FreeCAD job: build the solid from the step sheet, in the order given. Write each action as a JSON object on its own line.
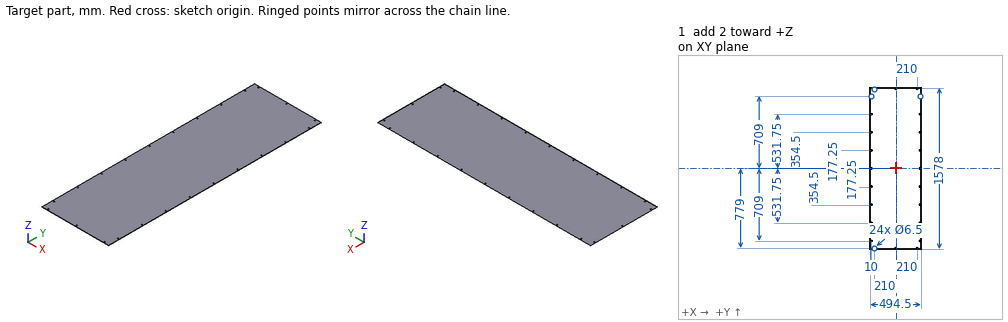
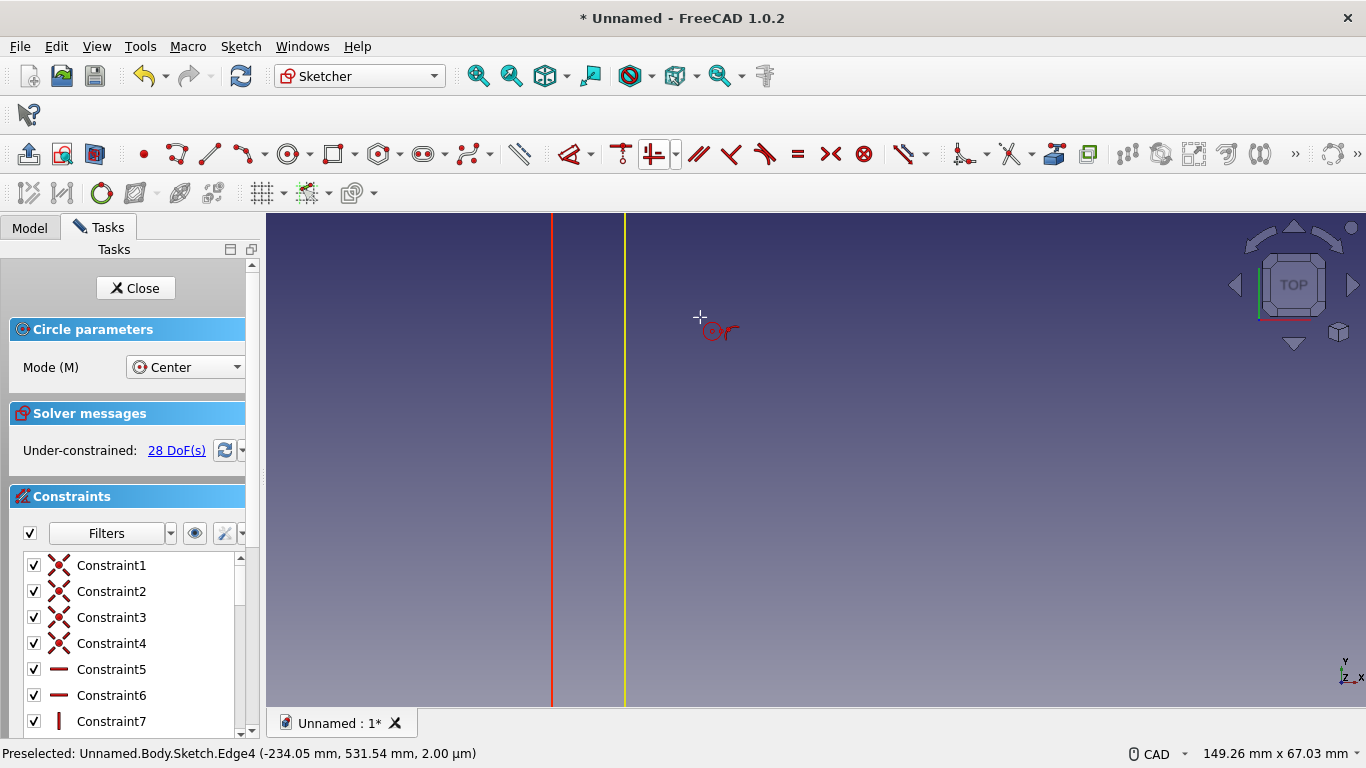
{"action": "scroll", "coordinate": [700, 317], "scroll_direction": "down", "scroll_amount": 18}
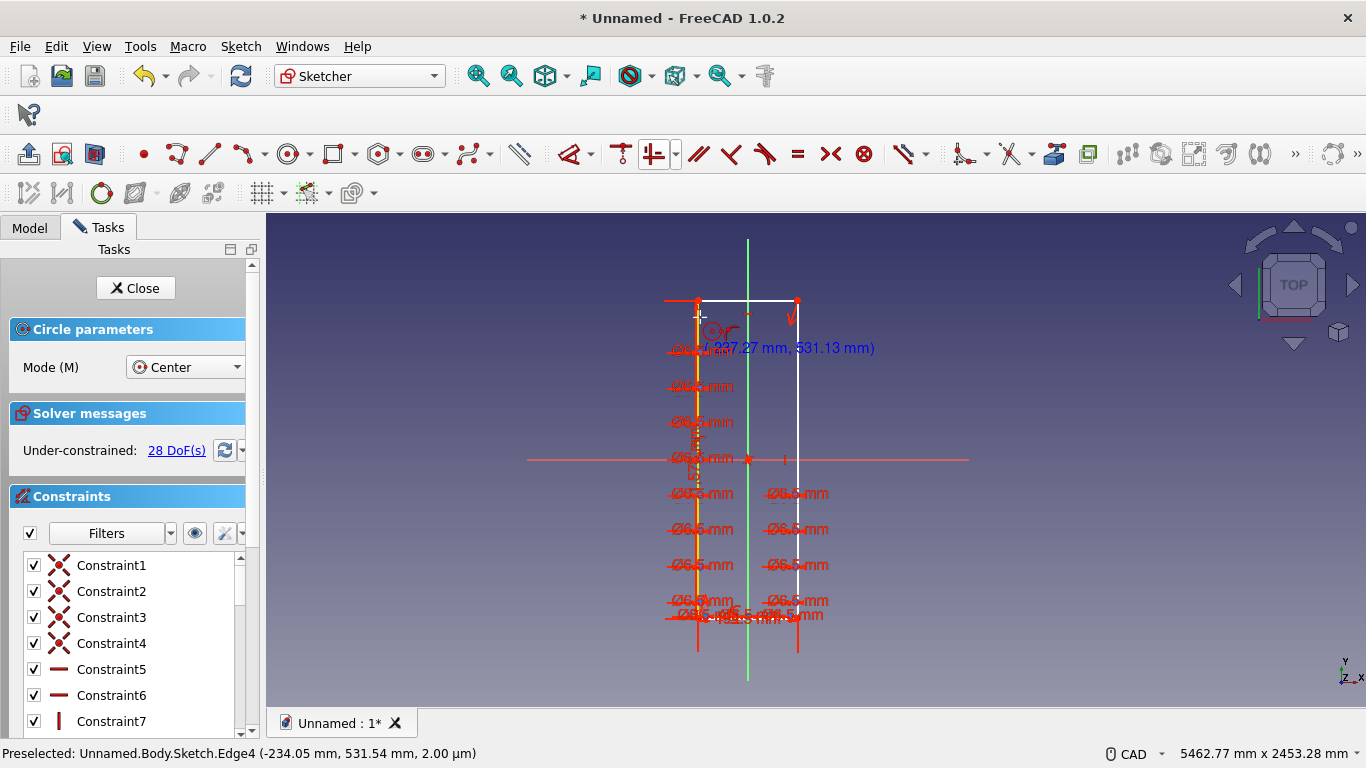
{"action": "scroll", "coordinate": [700, 317], "scroll_direction": "up", "scroll_amount": 11}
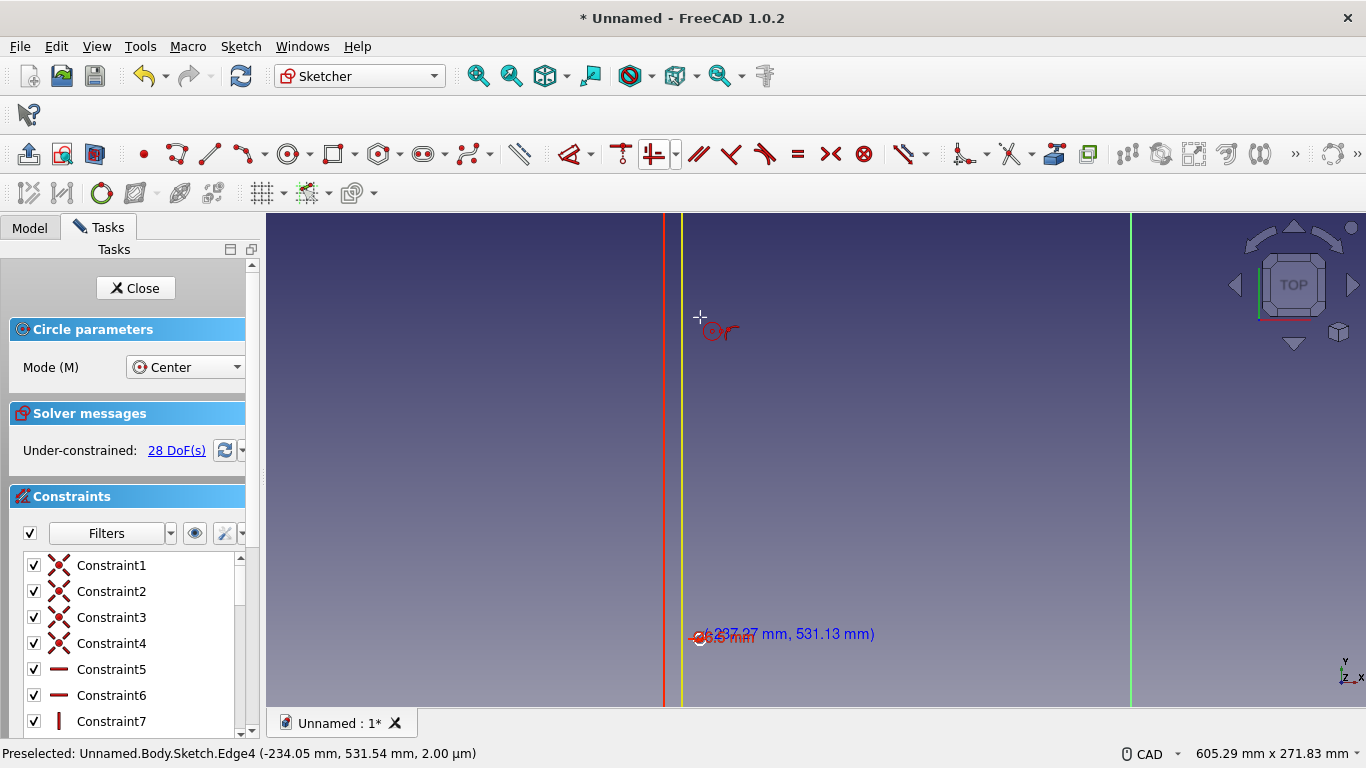
{"action": "left_click", "coordinate": [700, 316]}
{"action": "mouse_move", "coordinate": [704, 312]}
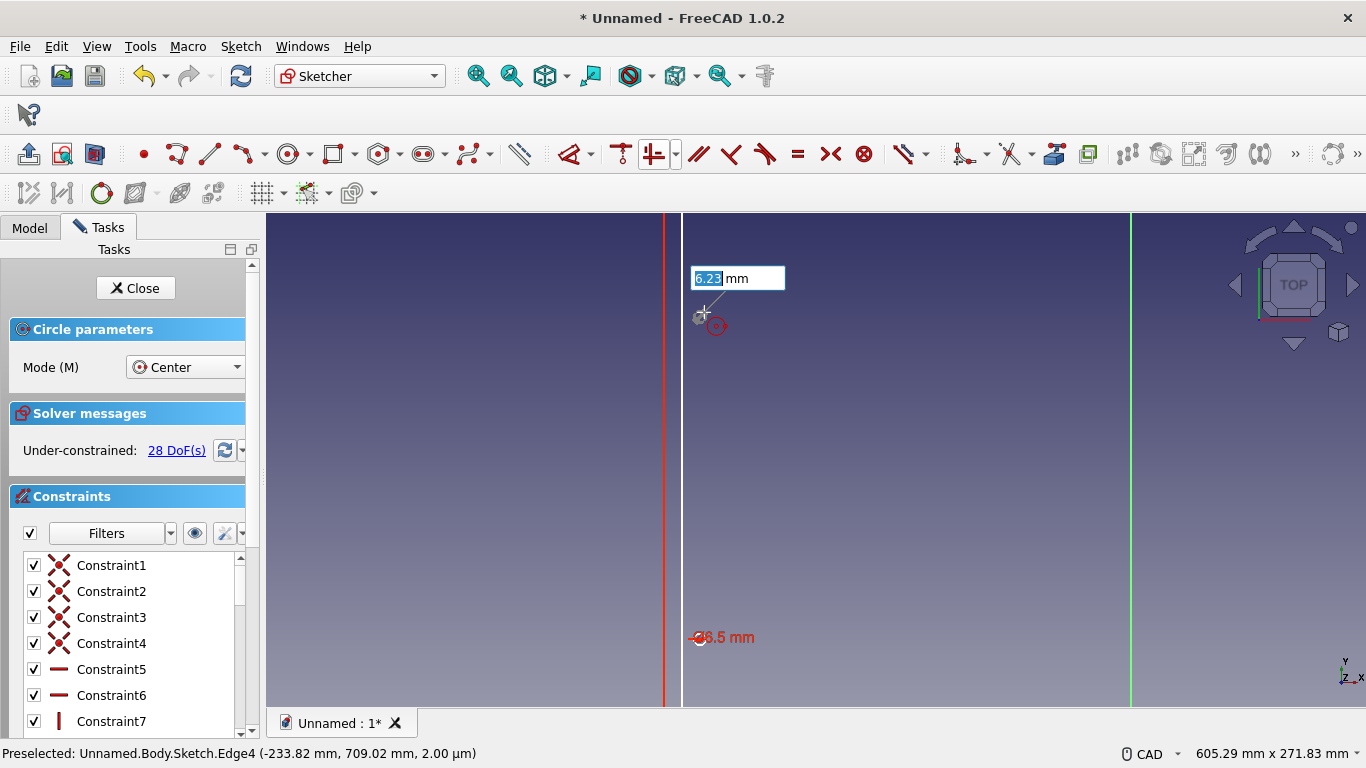
{"action": "type", "text": "6.5"}
{"action": "key", "text": "Return"}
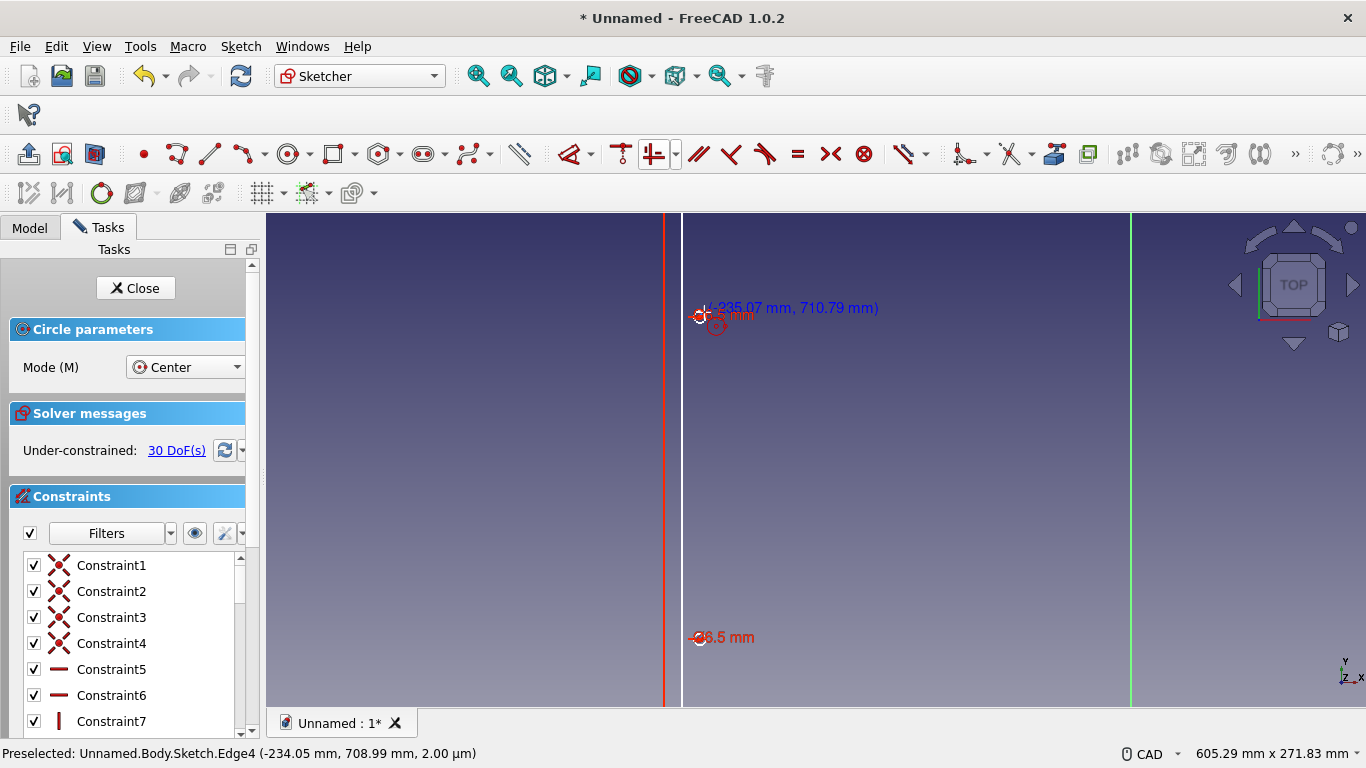
{"action": "scroll", "coordinate": [700, 317], "scroll_direction": "down", "scroll_amount": 11}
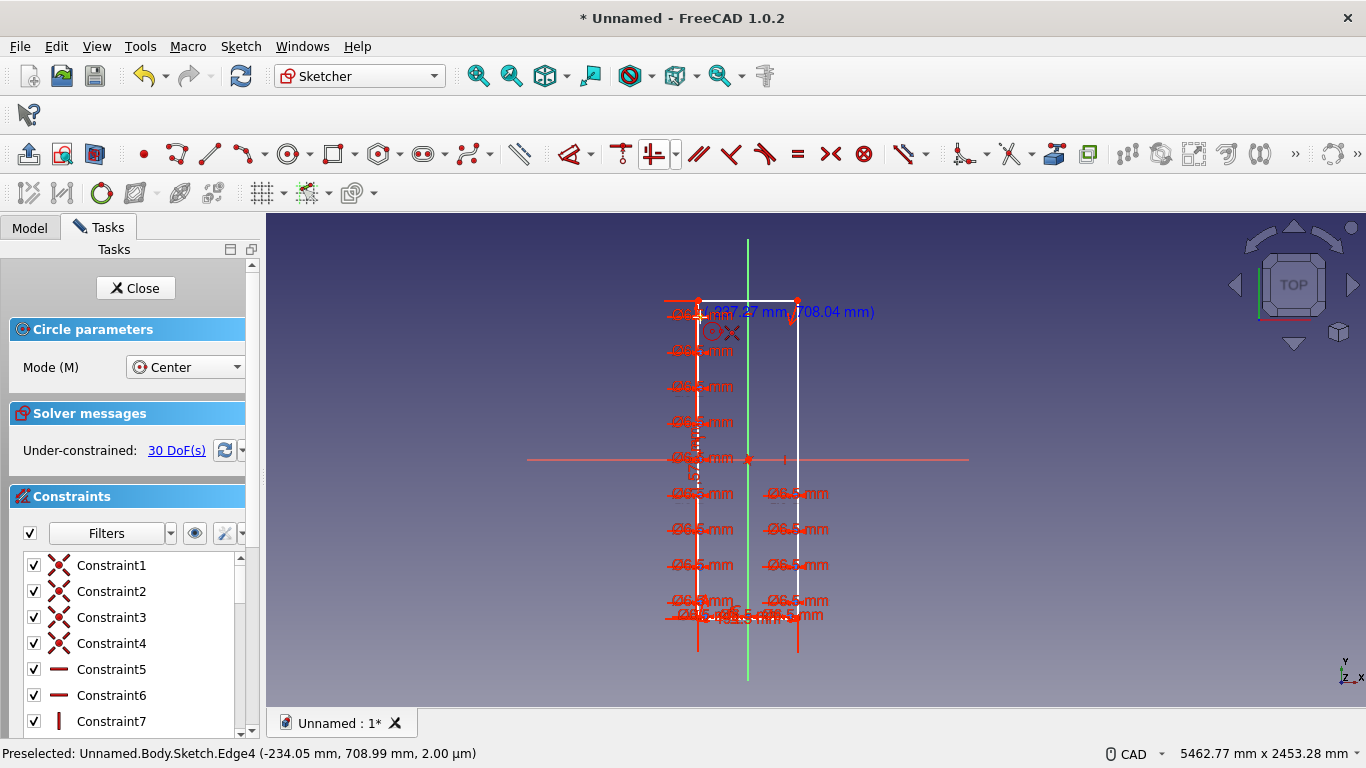
{"action": "scroll", "coordinate": [706, 303], "scroll_direction": "up", "scroll_amount": 18}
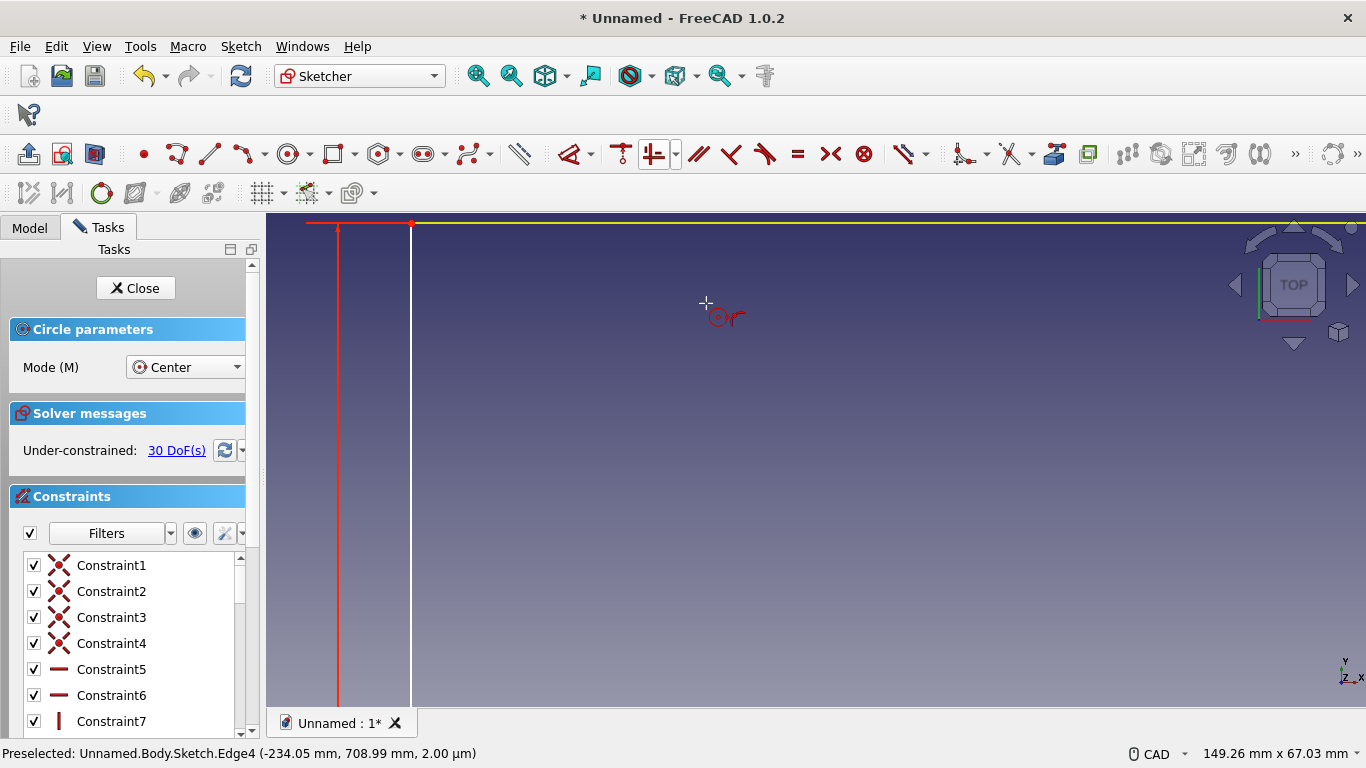
{"action": "scroll", "coordinate": [706, 303], "scroll_direction": "down", "scroll_amount": 18}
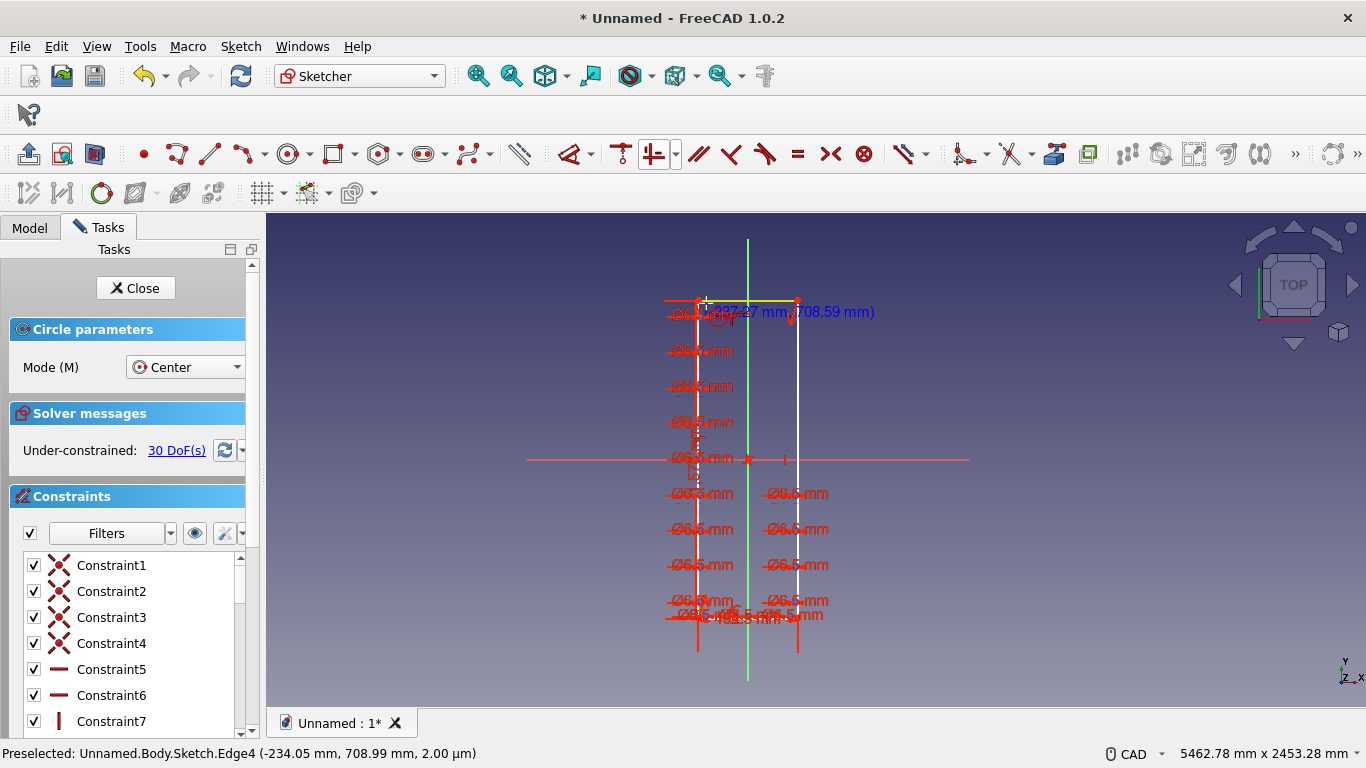
{"action": "scroll", "coordinate": [706, 303], "scroll_direction": "up", "scroll_amount": 11}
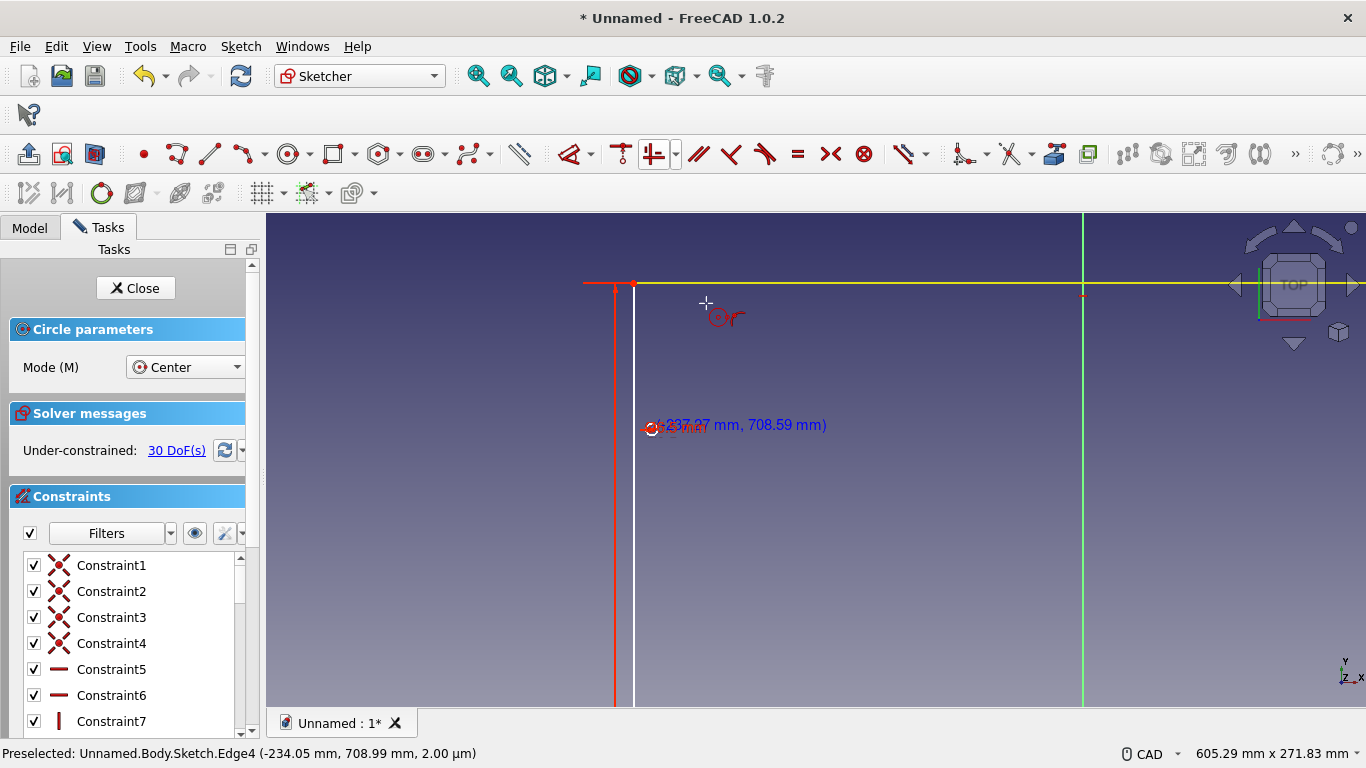
{"action": "left_click", "coordinate": [701, 302]}
{"action": "mouse_move", "coordinate": [706, 306]}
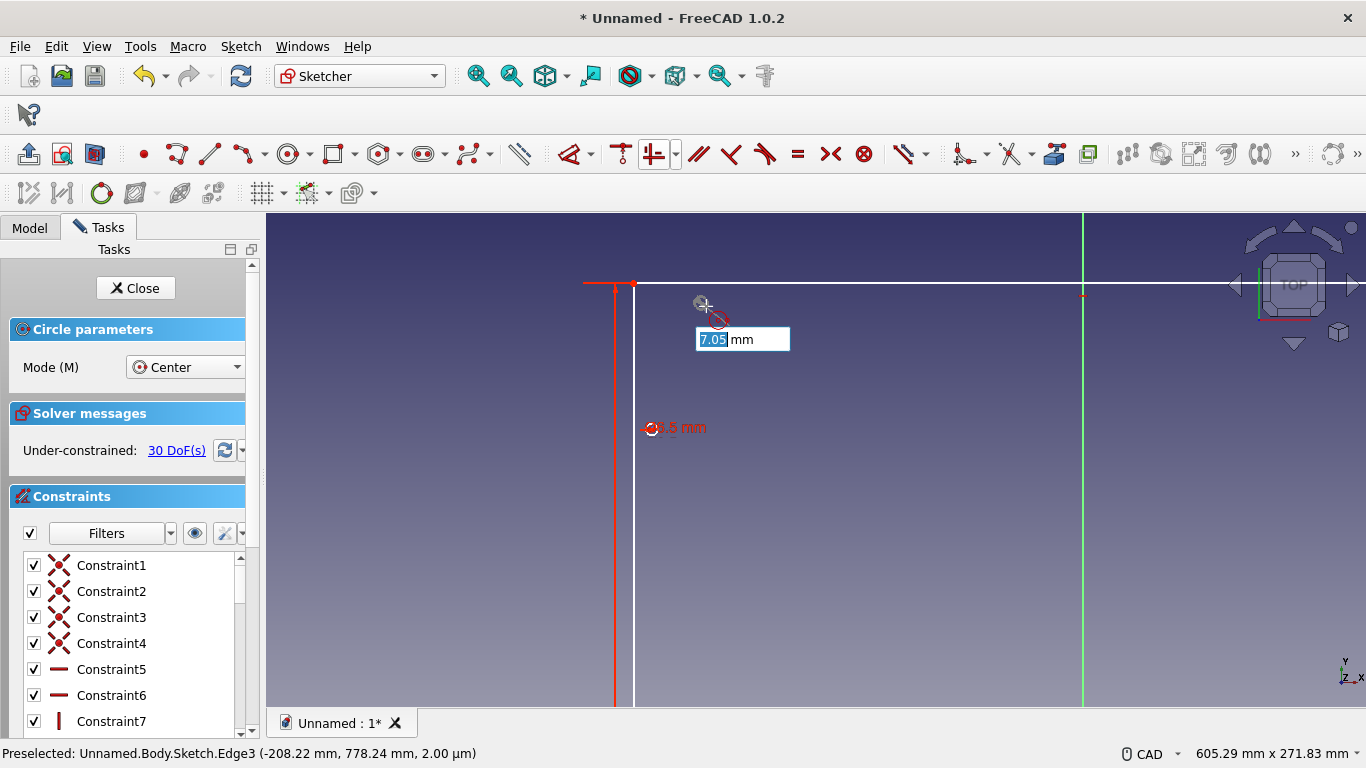
{"action": "type", "text": "6.5"}
{"action": "key", "text": "Return"}